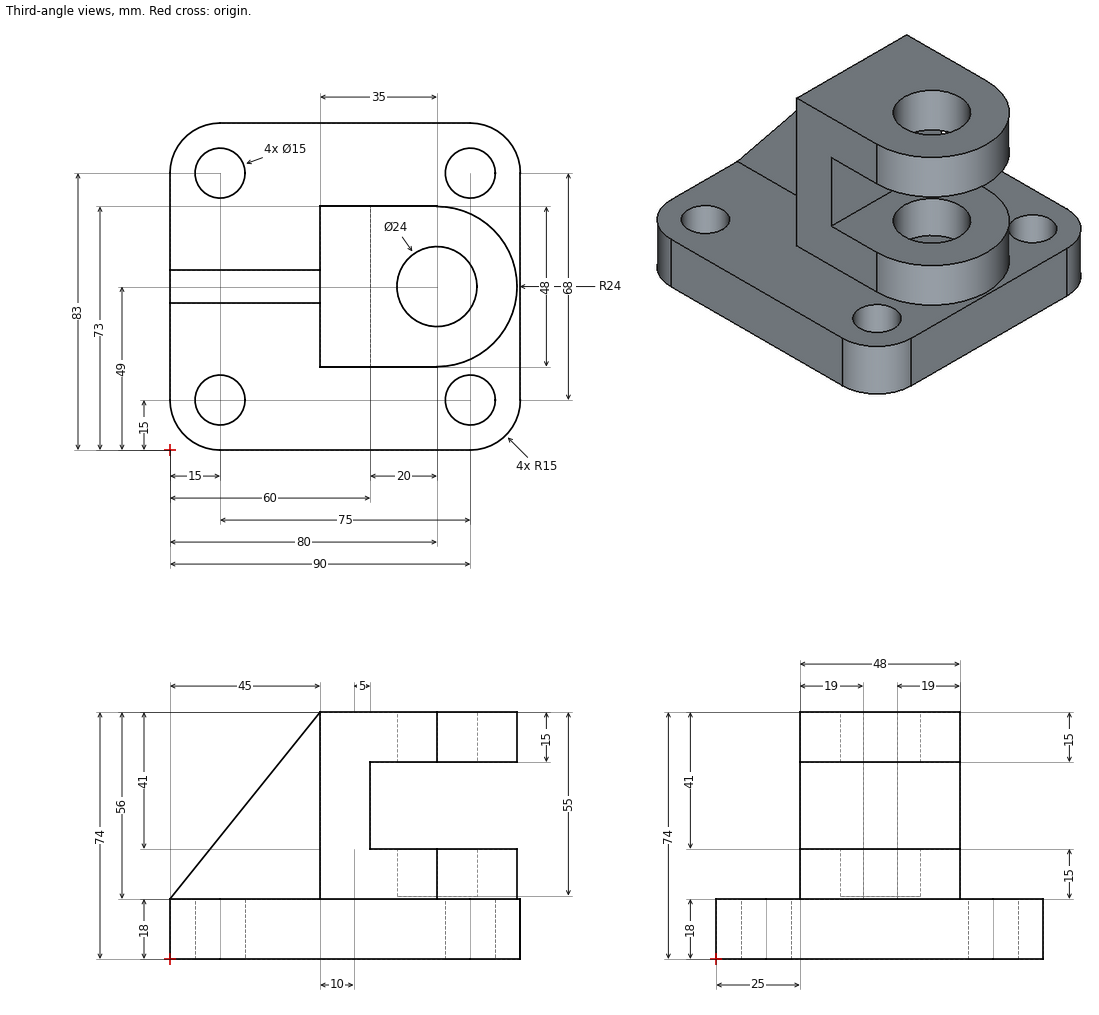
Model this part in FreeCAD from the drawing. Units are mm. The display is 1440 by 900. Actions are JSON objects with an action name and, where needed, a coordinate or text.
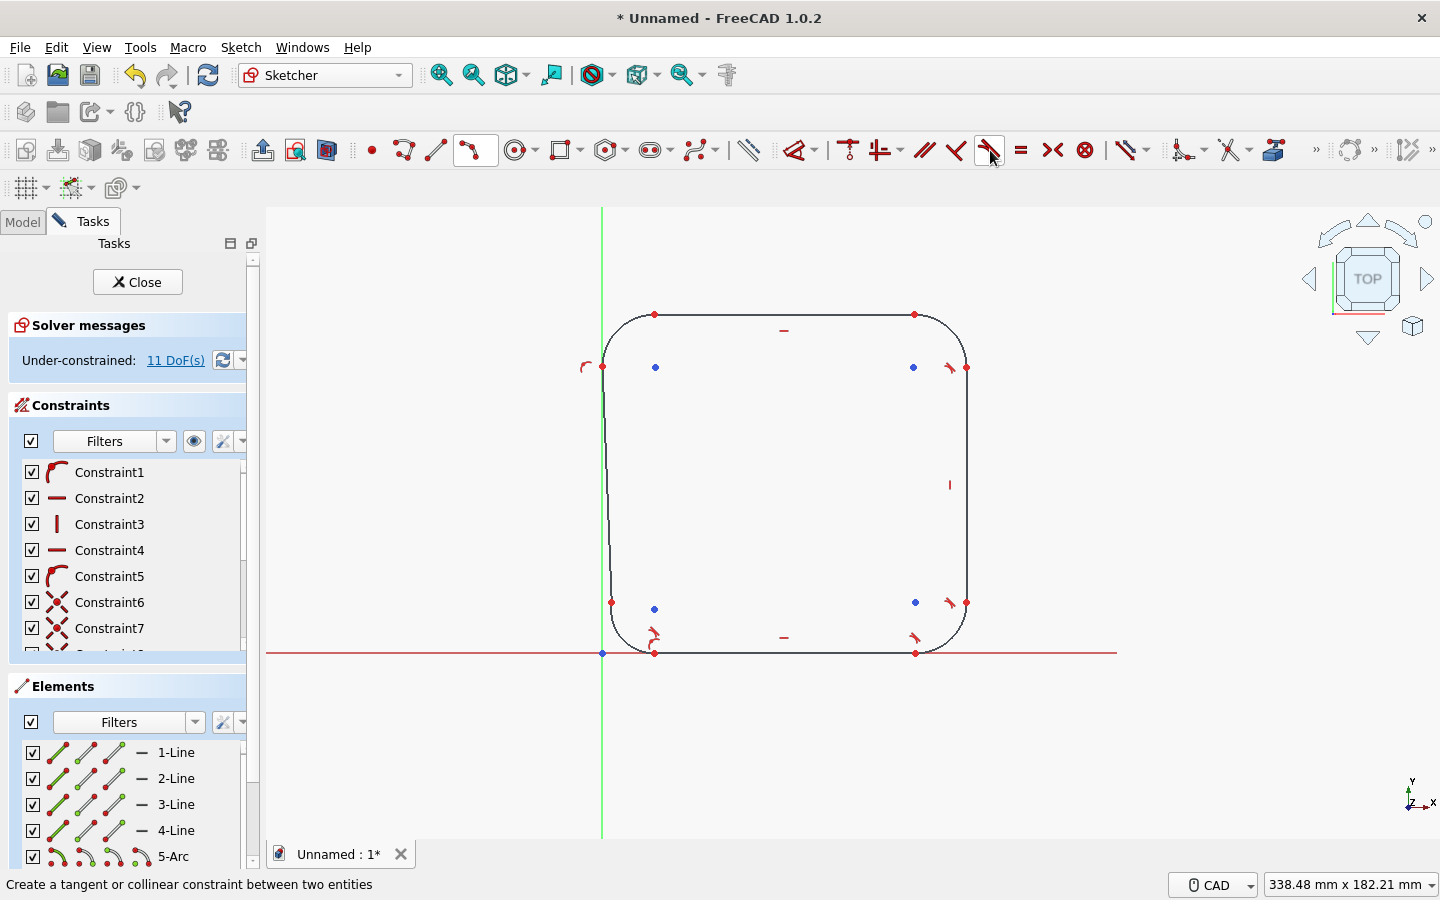
{"action": "left_click", "coordinate": [837, 315]}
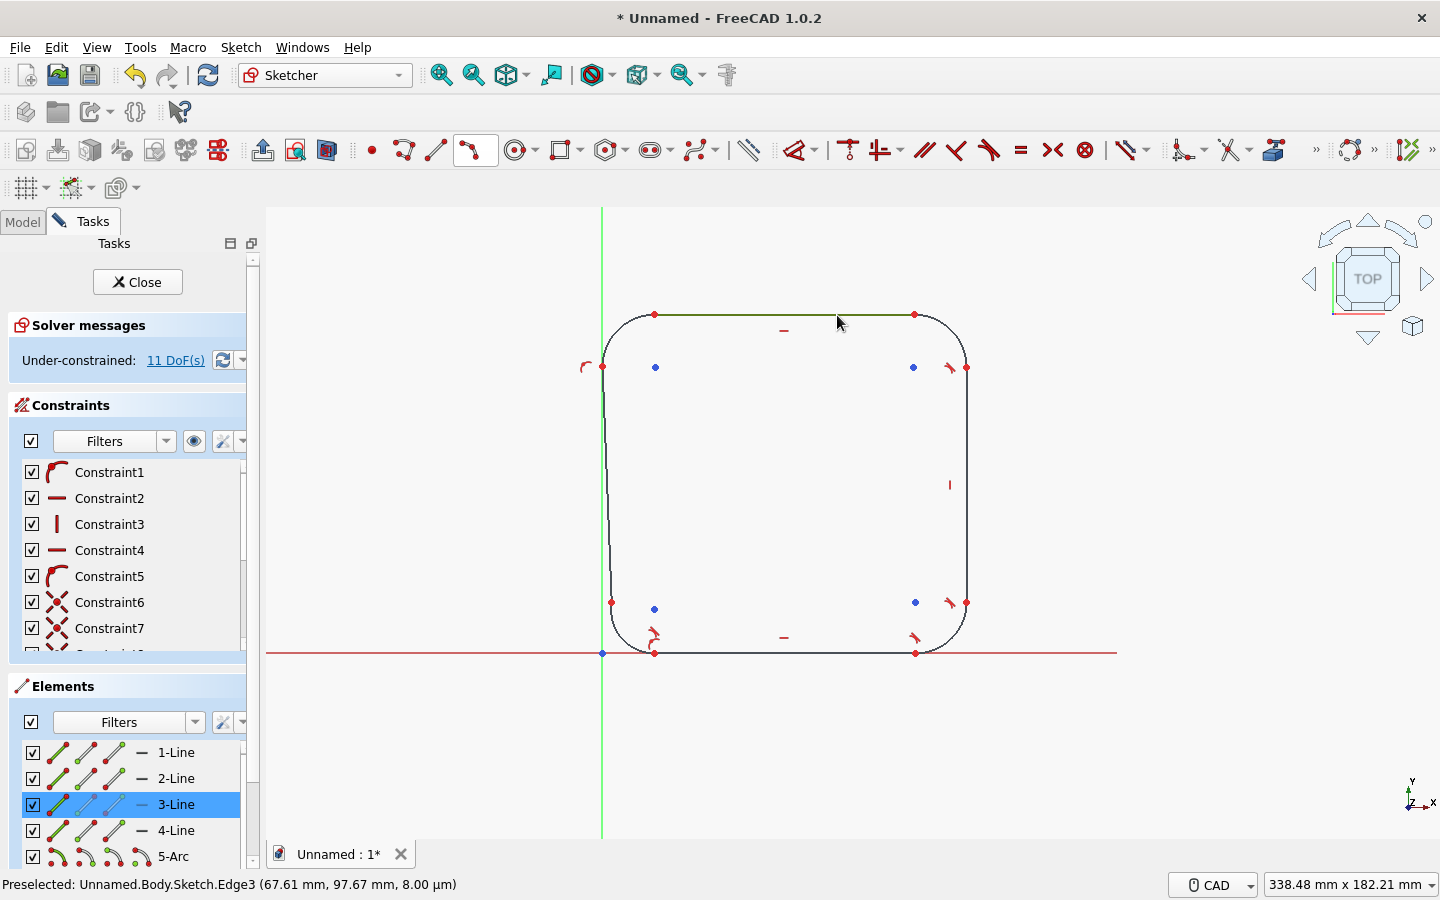
{"action": "left_click", "coordinate": [961, 344]}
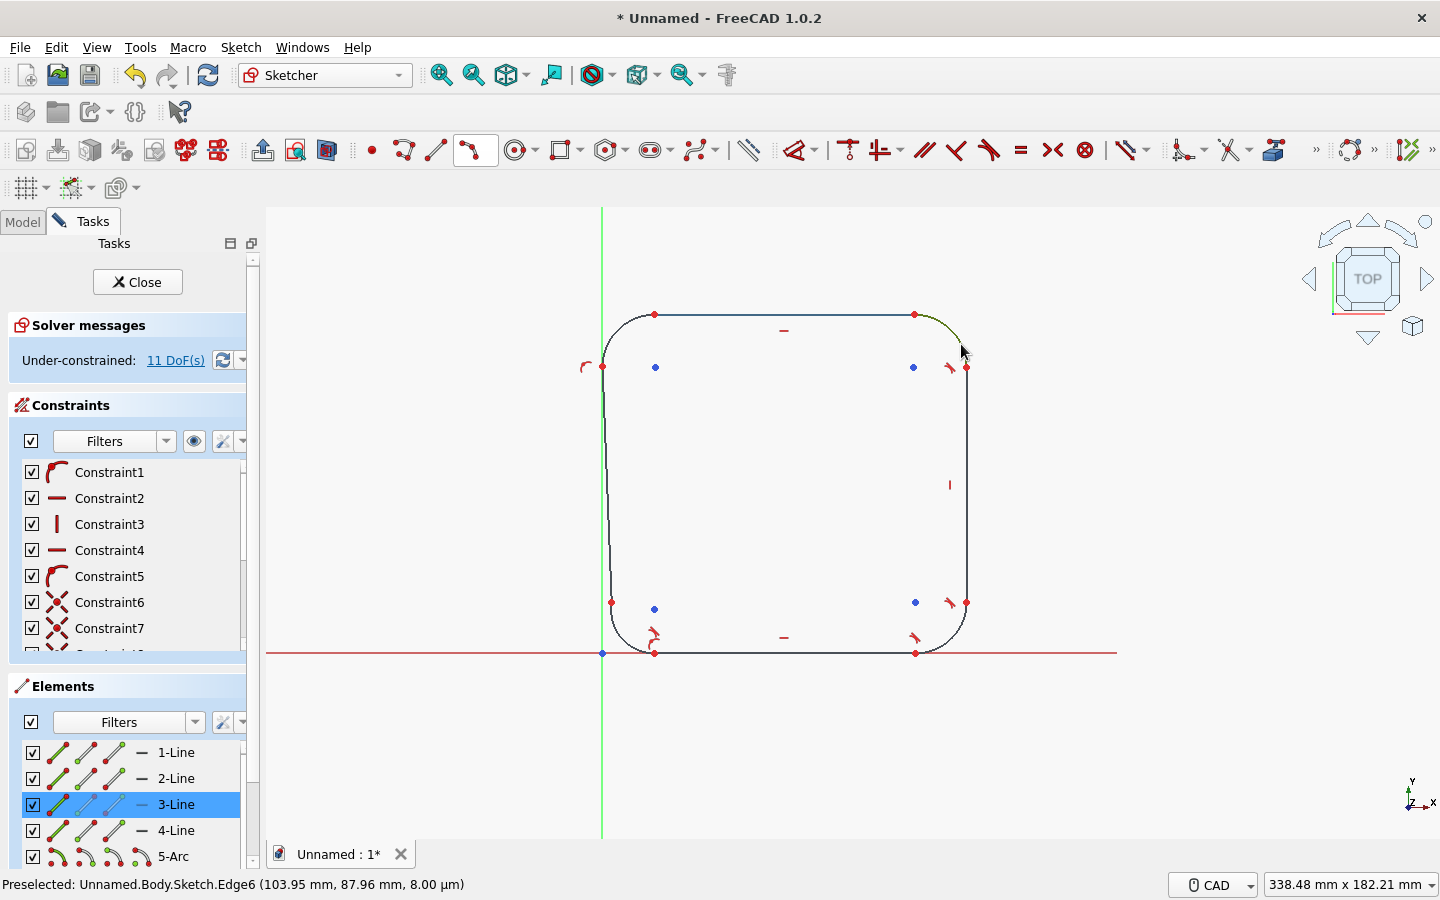
{"action": "left_click", "coordinate": [990, 150]}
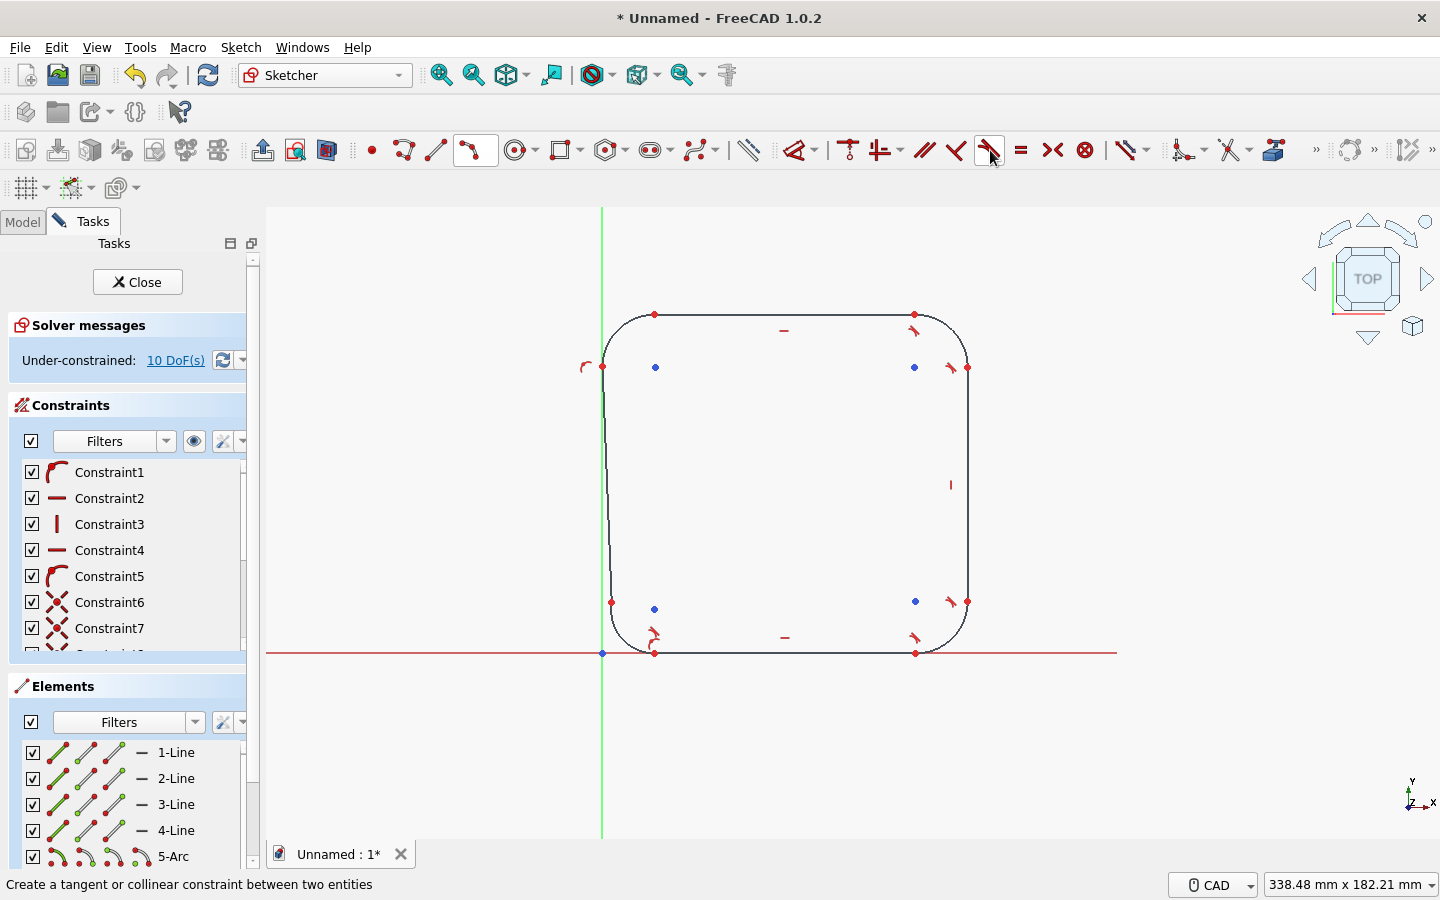
{"action": "left_click", "coordinate": [837, 315]}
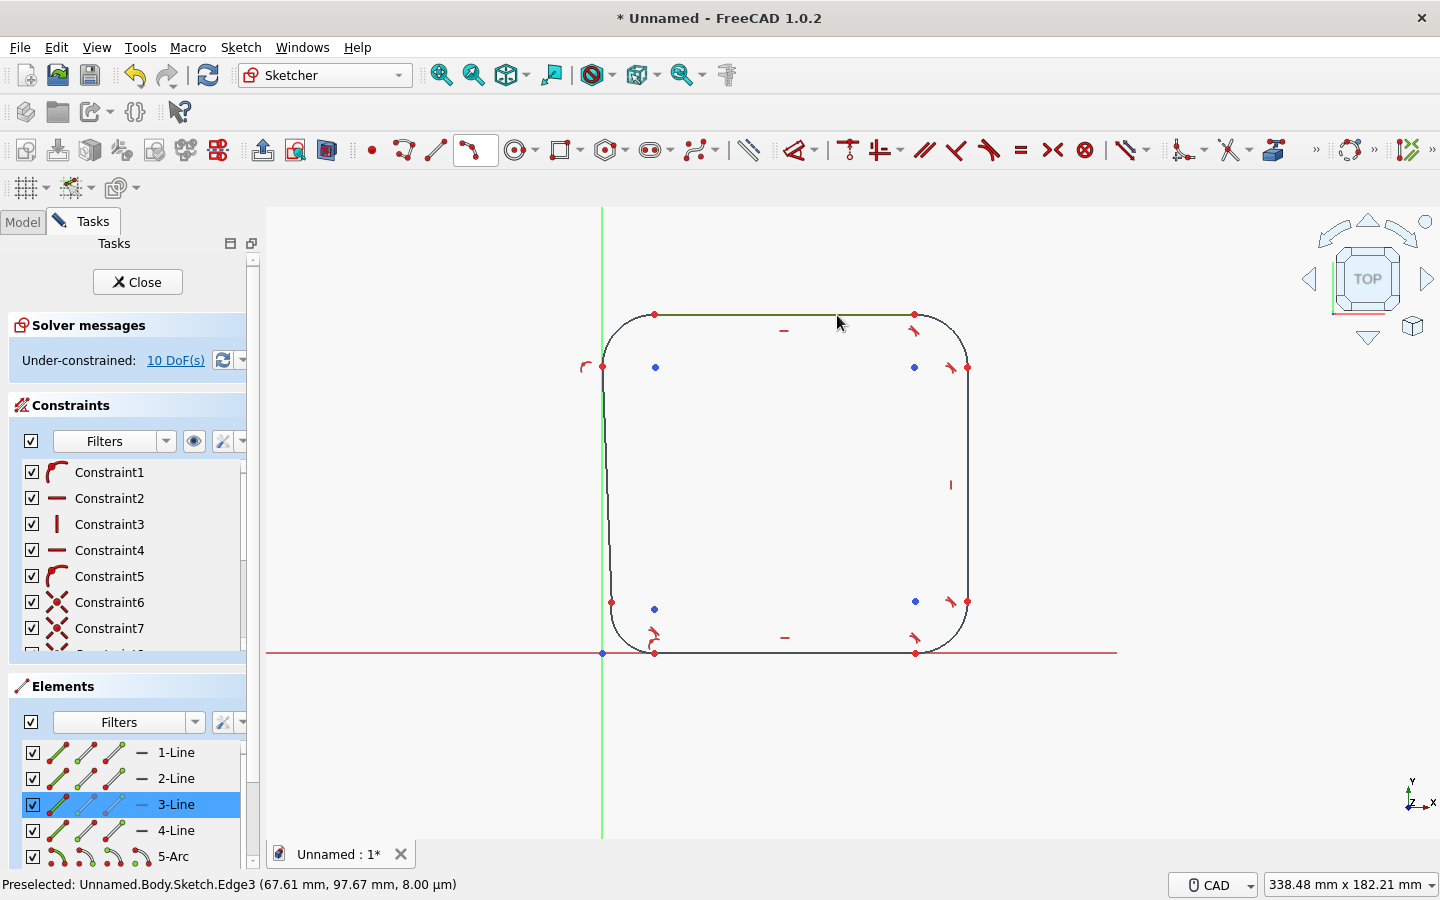
{"action": "left_click", "coordinate": [631, 320]}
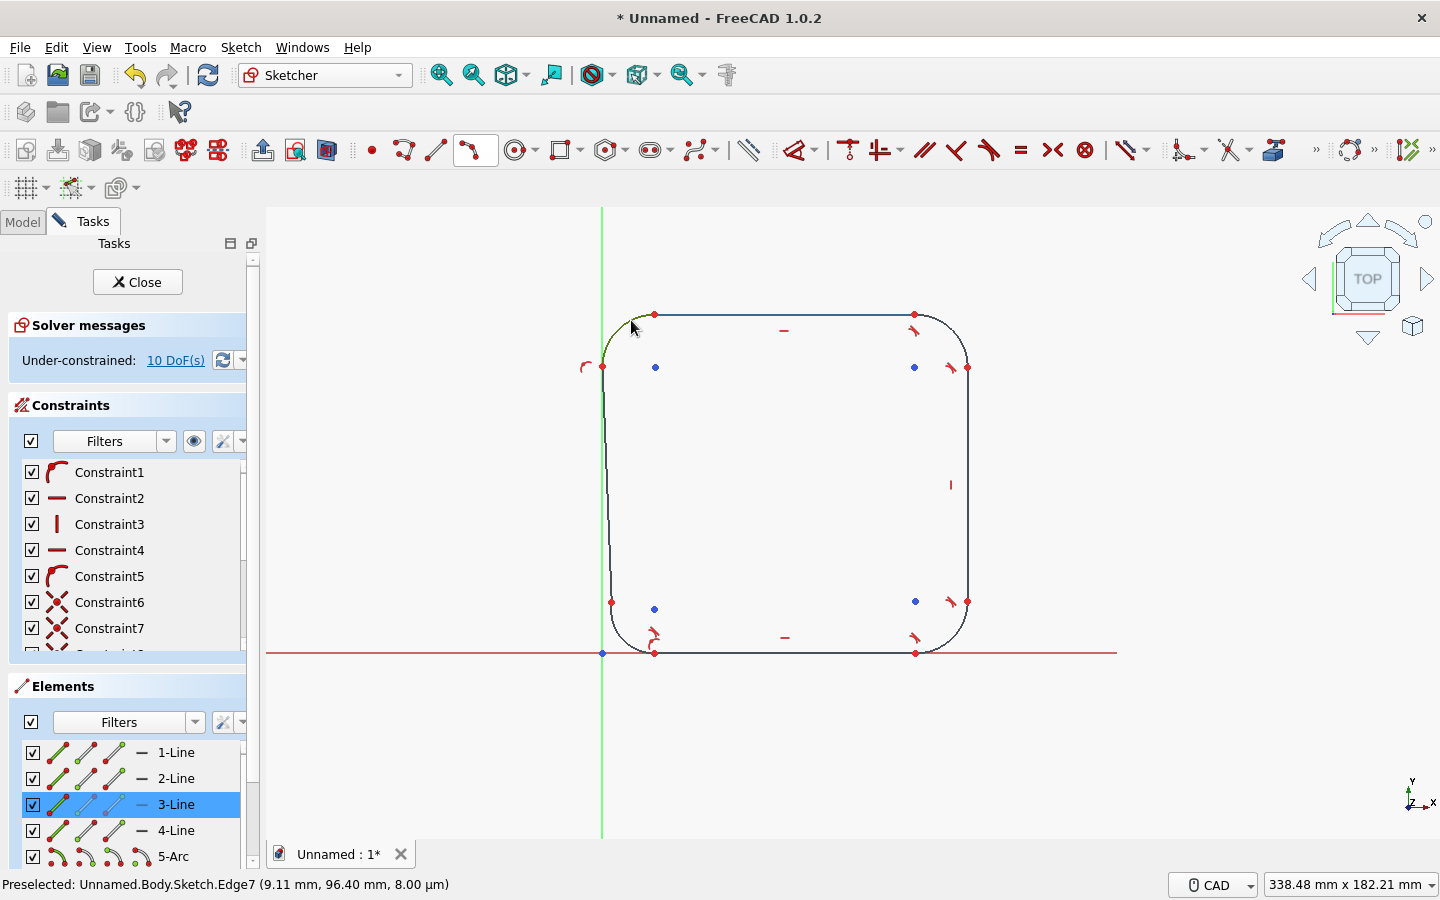
{"action": "left_click", "coordinate": [990, 150]}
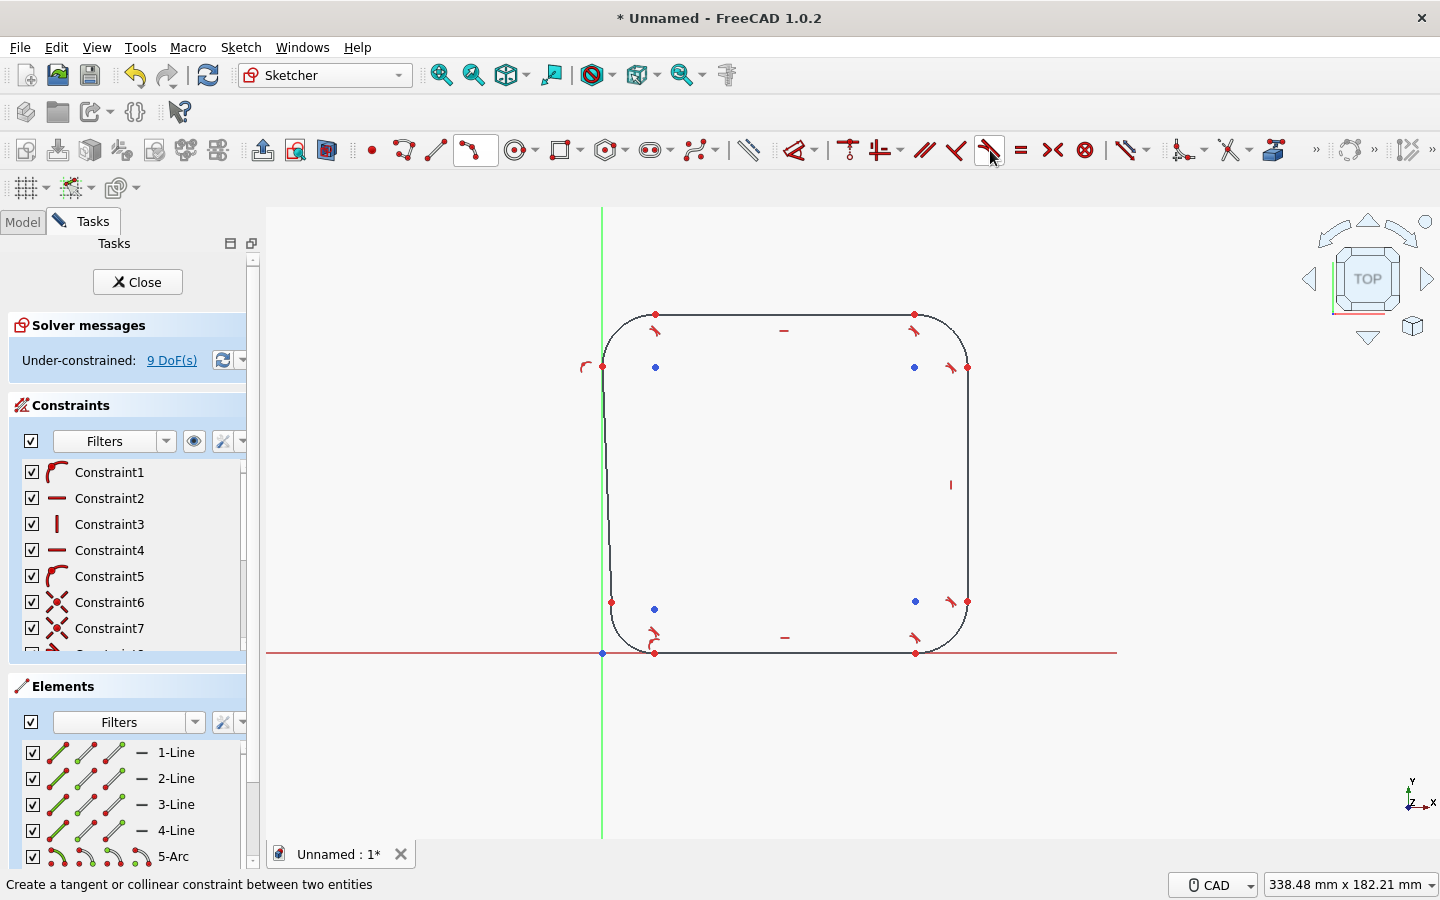
{"action": "left_click", "coordinate": [605, 437]}